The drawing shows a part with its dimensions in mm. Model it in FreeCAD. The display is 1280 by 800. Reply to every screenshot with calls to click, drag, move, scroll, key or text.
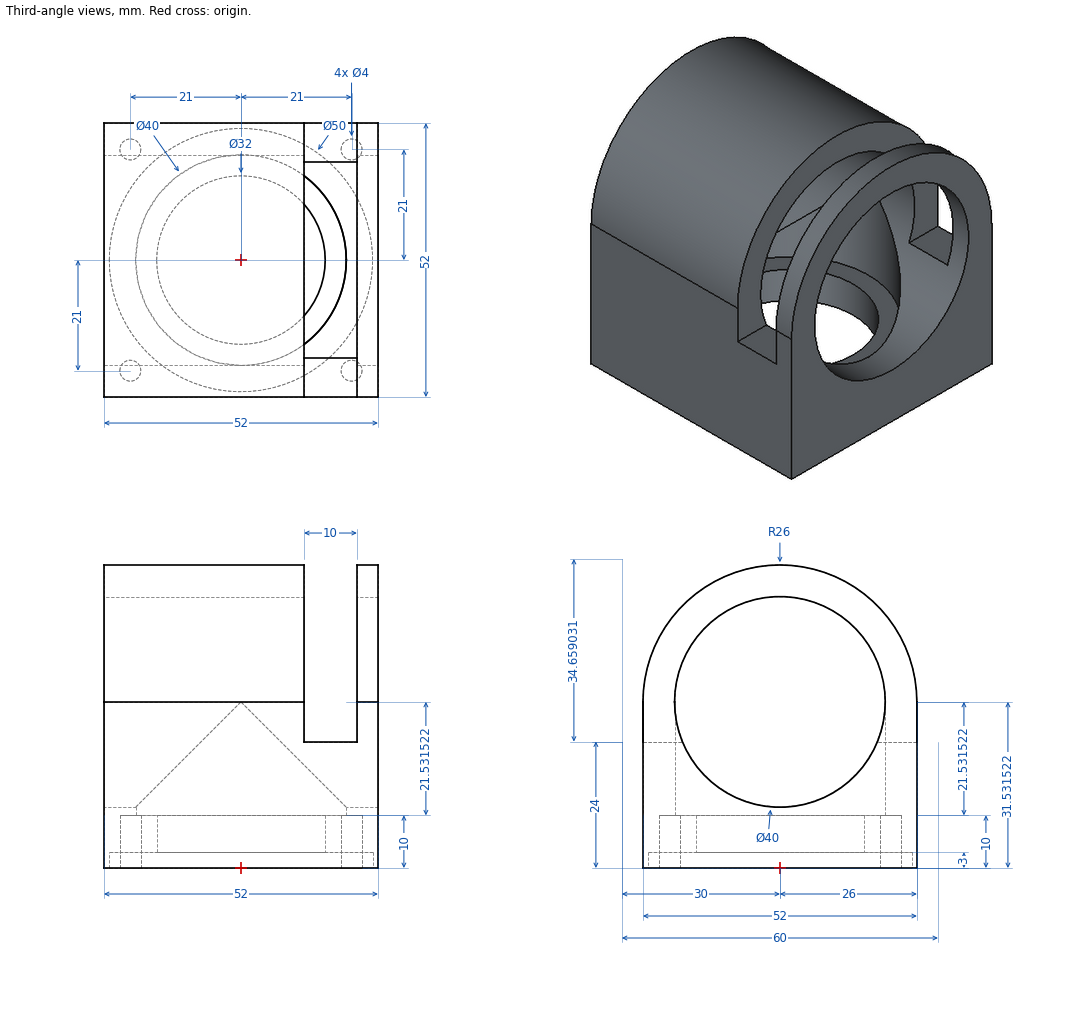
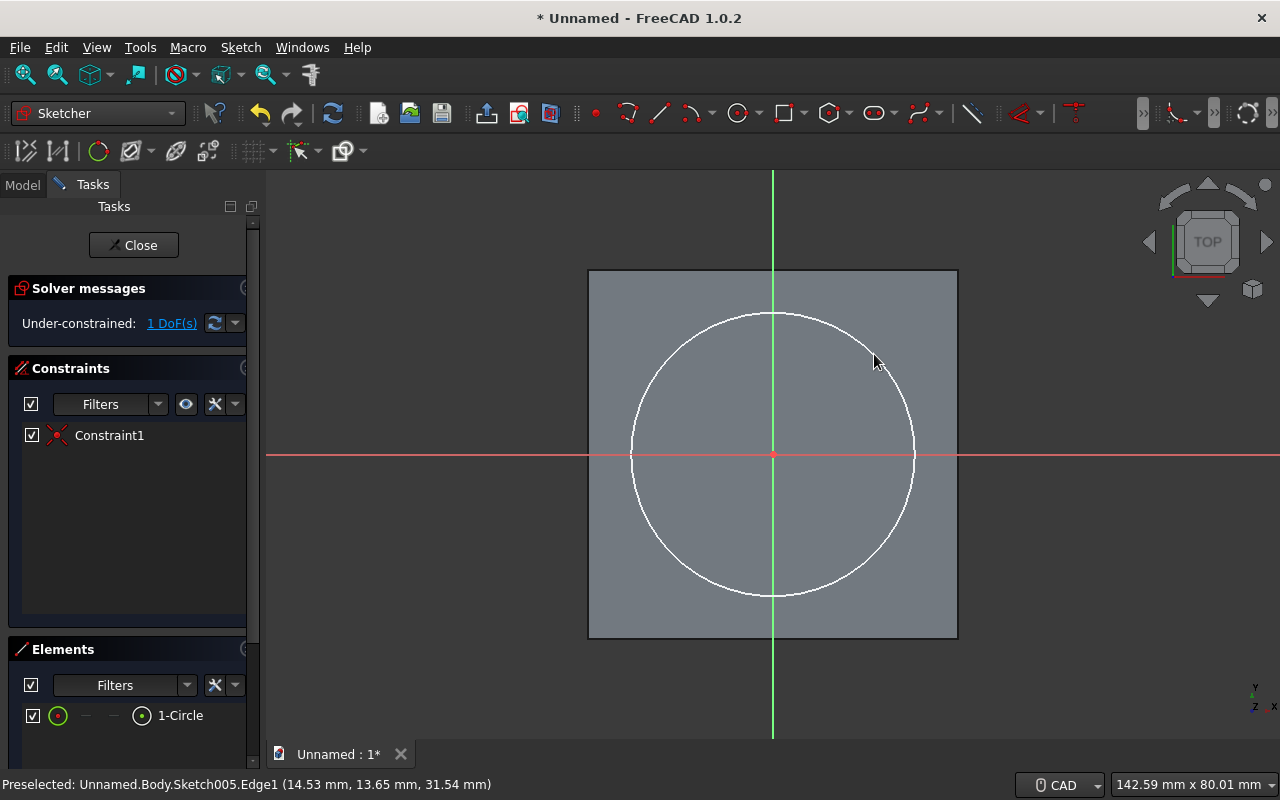
click(1020, 114)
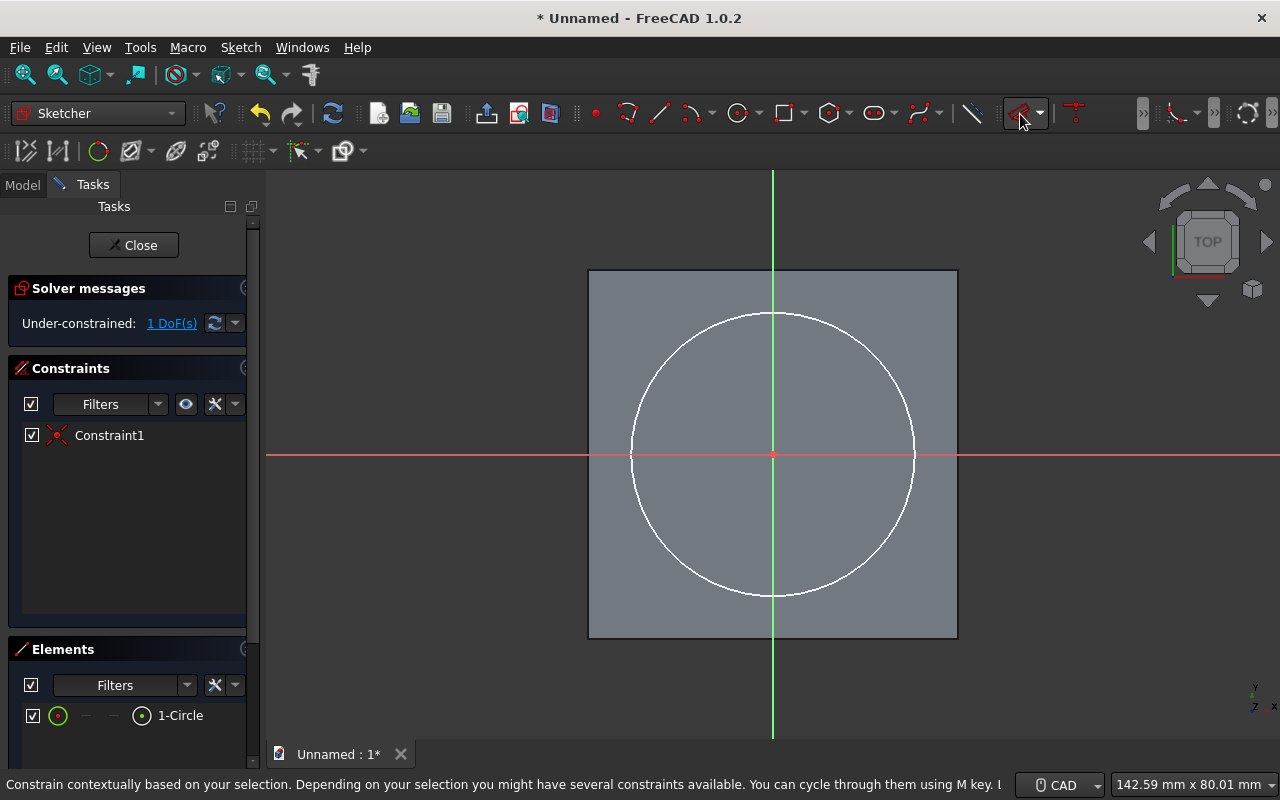
click(873, 354)
click(896, 331)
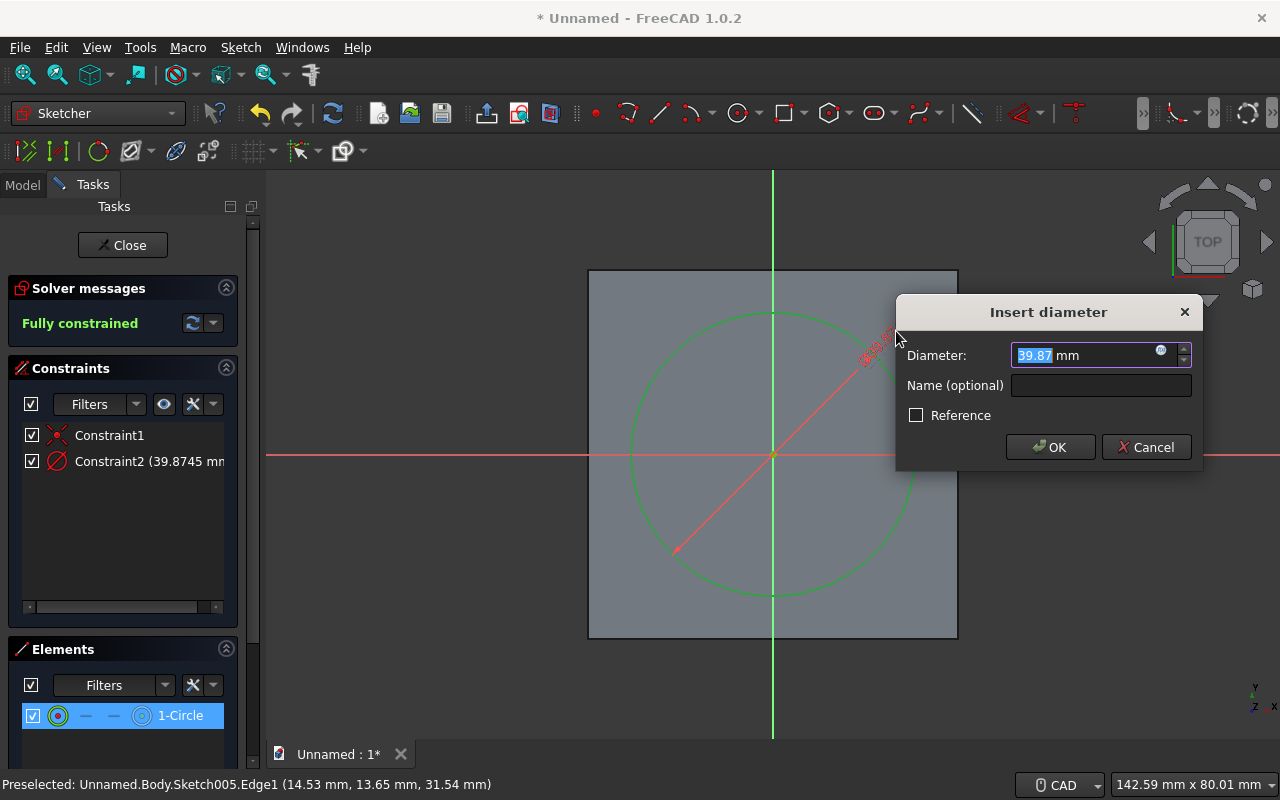
text(40)
key(Return)
key(Escape)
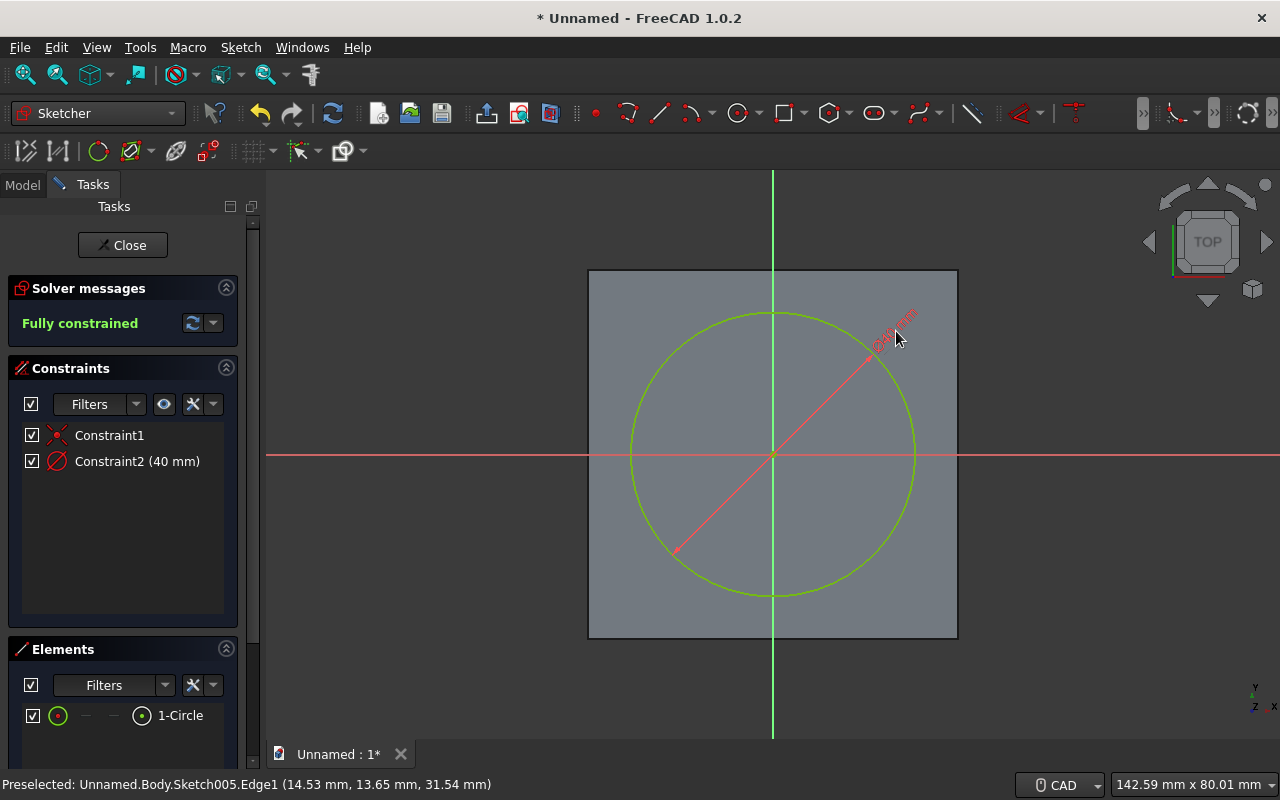
click(123, 245)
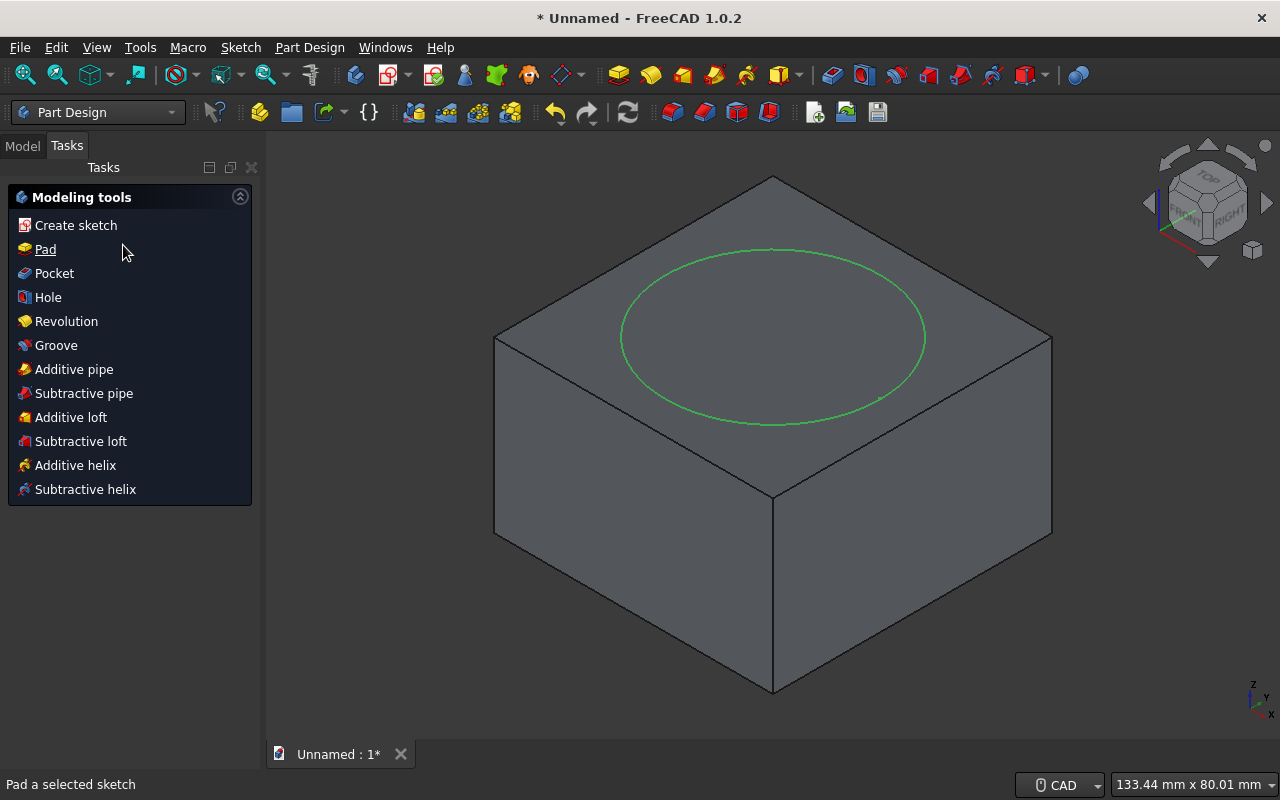
click(834, 76)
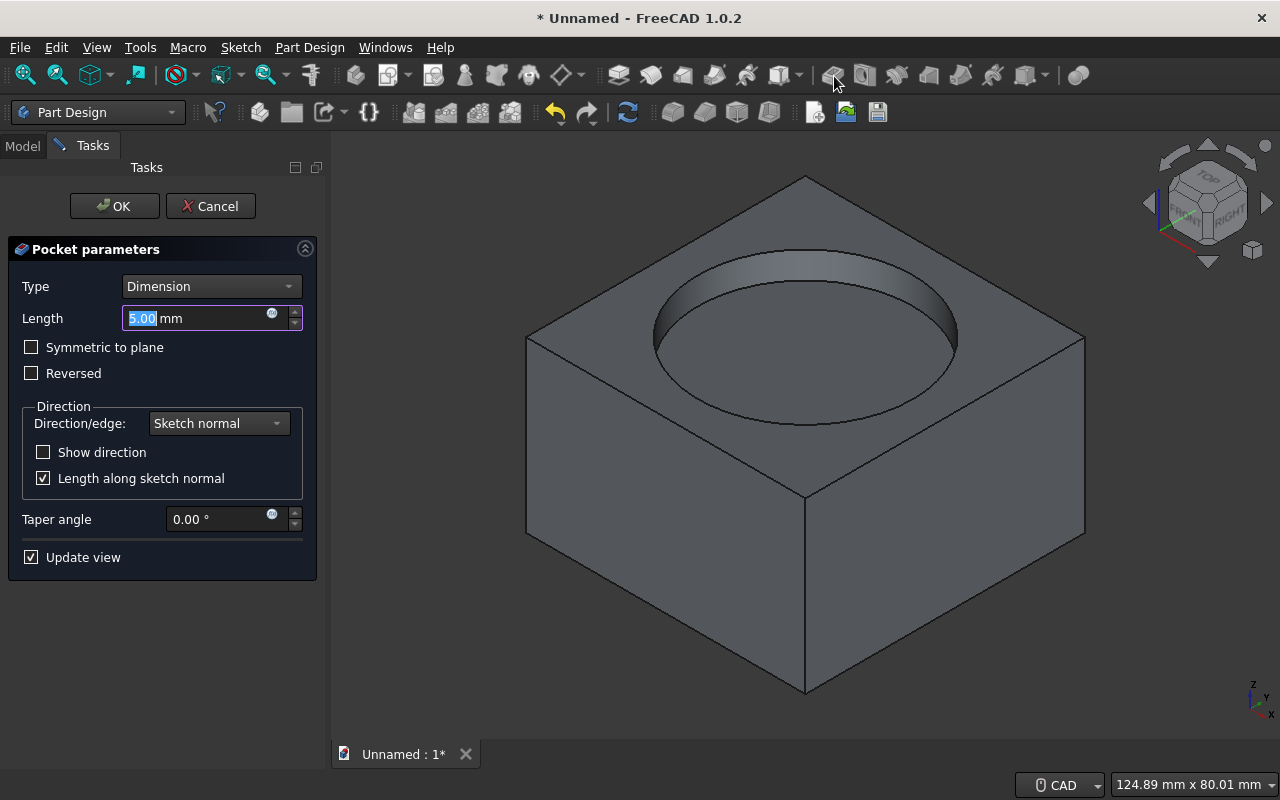
text(21.531522)
key(Tab)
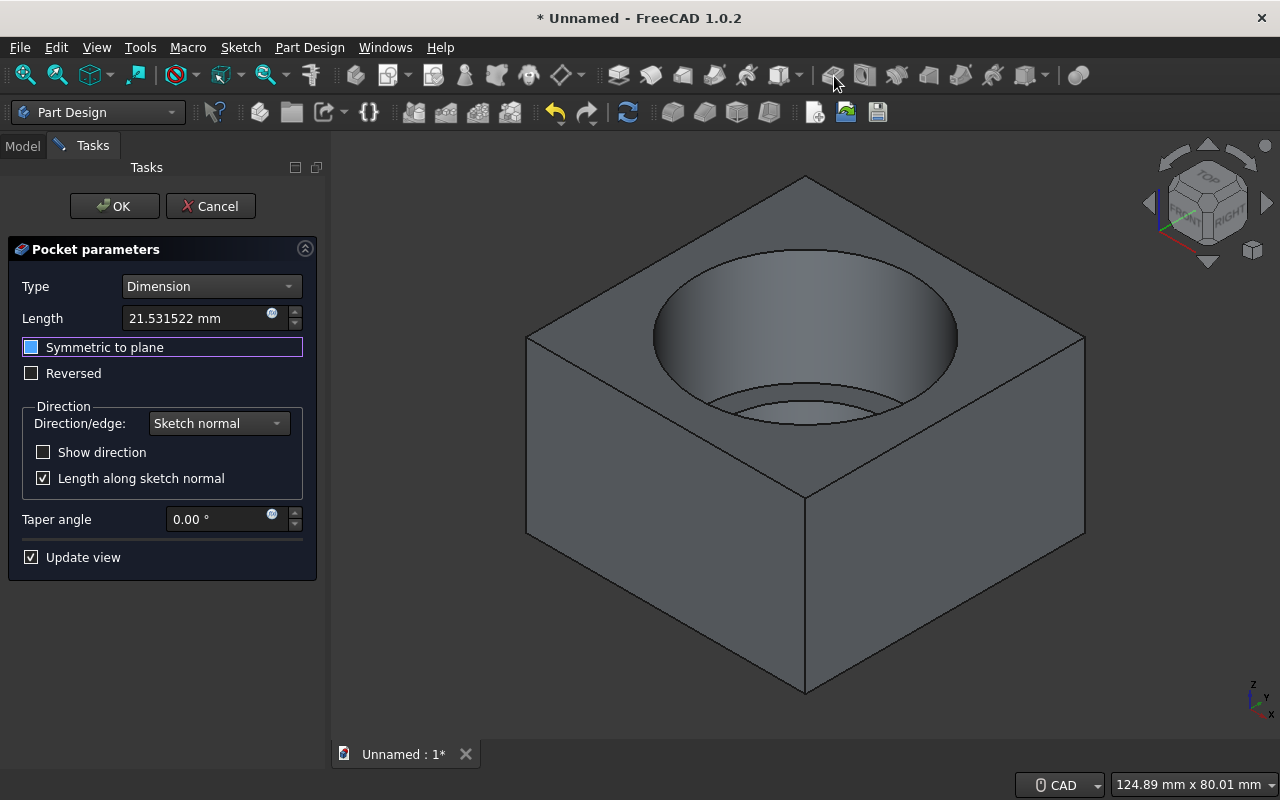
click(115, 206)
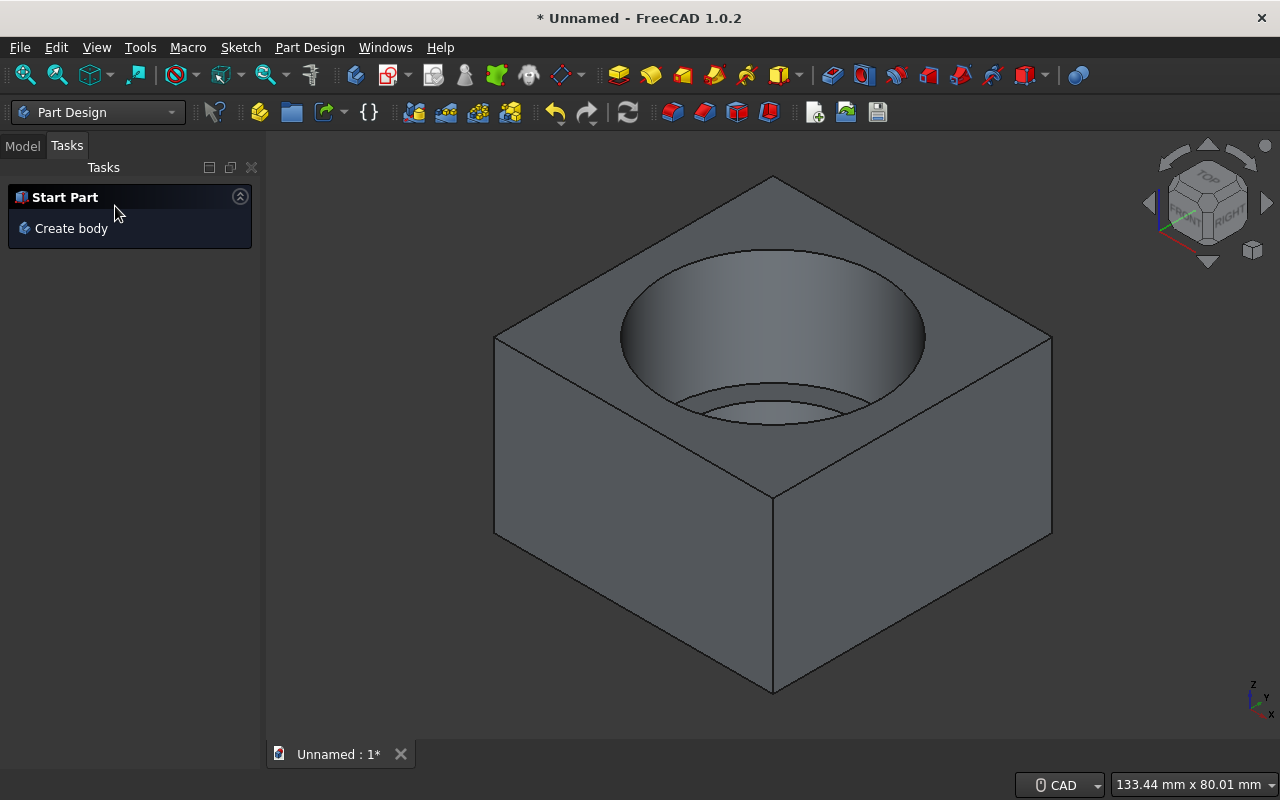
key(6)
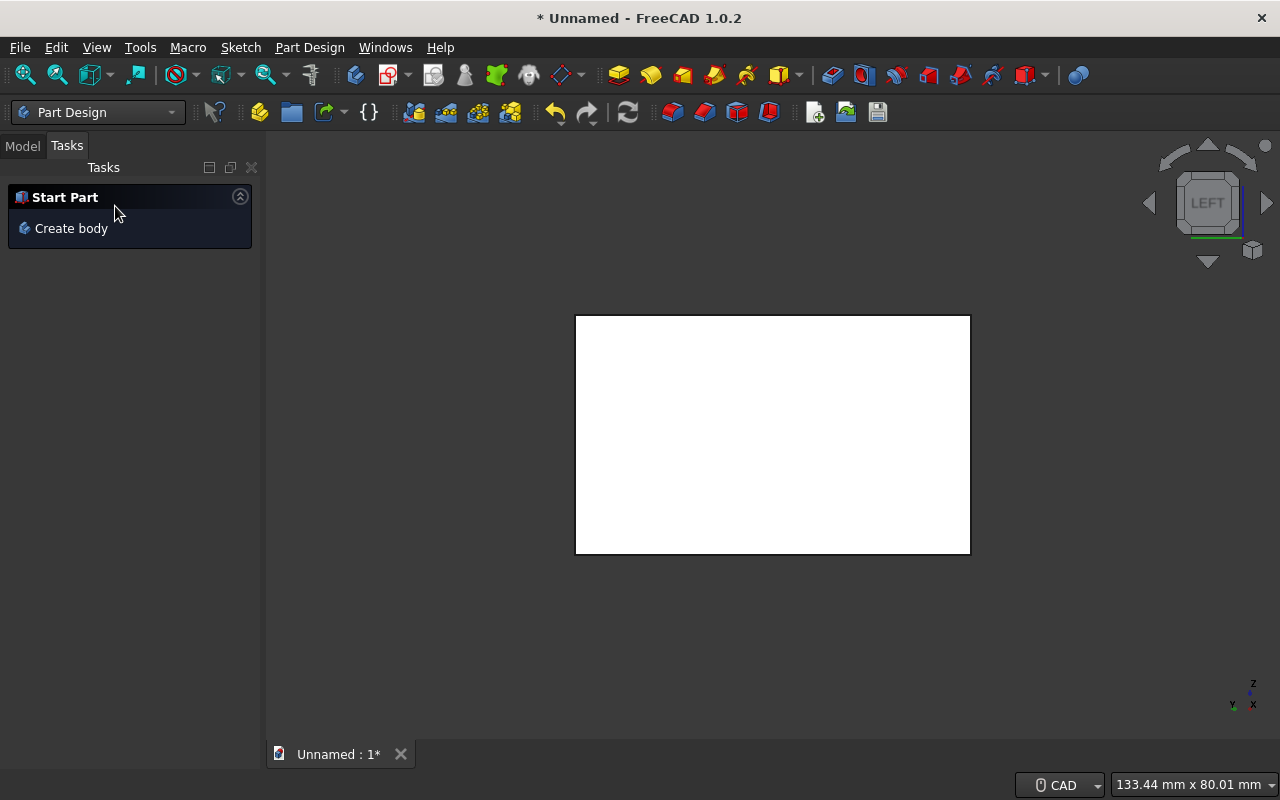
click(26, 76)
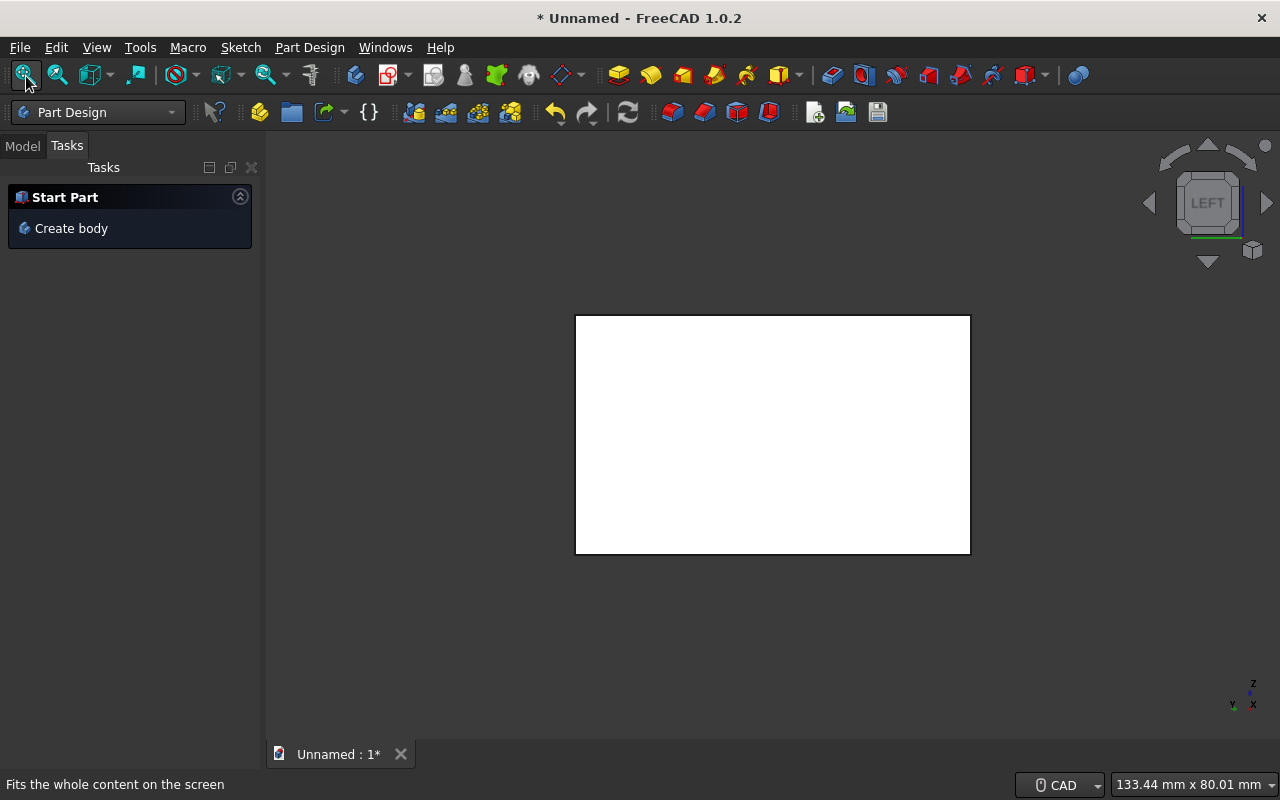
click(717, 434)